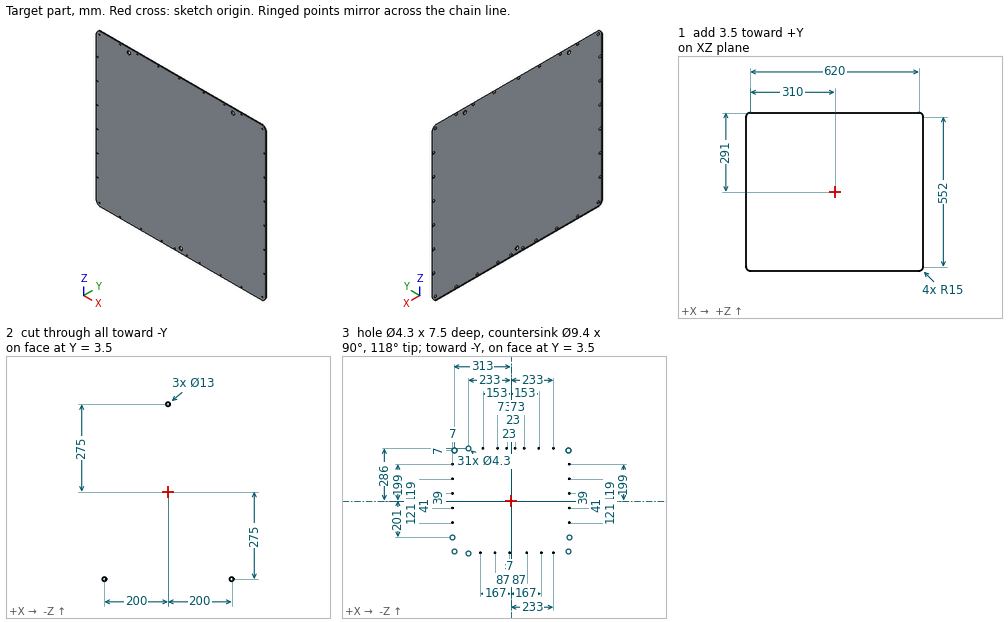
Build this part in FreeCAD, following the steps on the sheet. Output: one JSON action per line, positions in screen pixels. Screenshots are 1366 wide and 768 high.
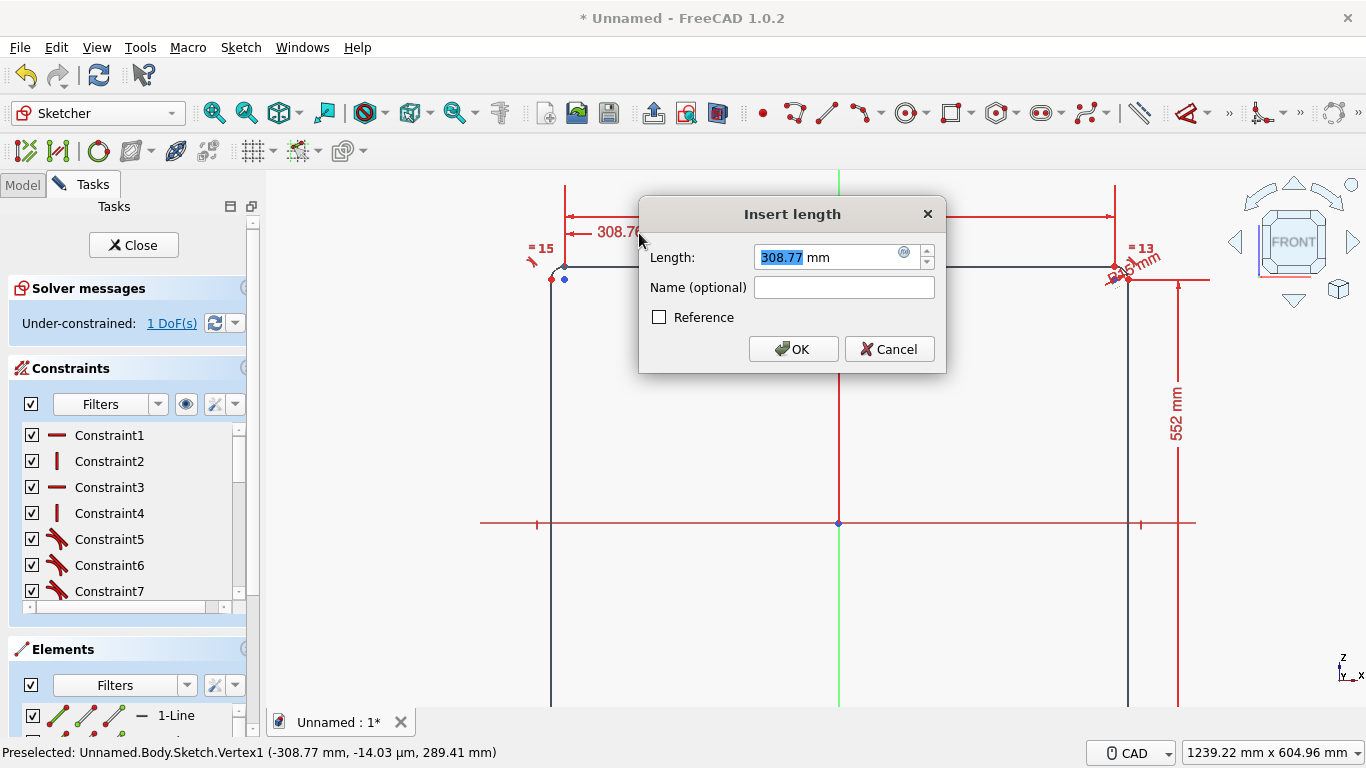
{"action": "type", "text": "310"}
{"action": "key", "text": "Return"}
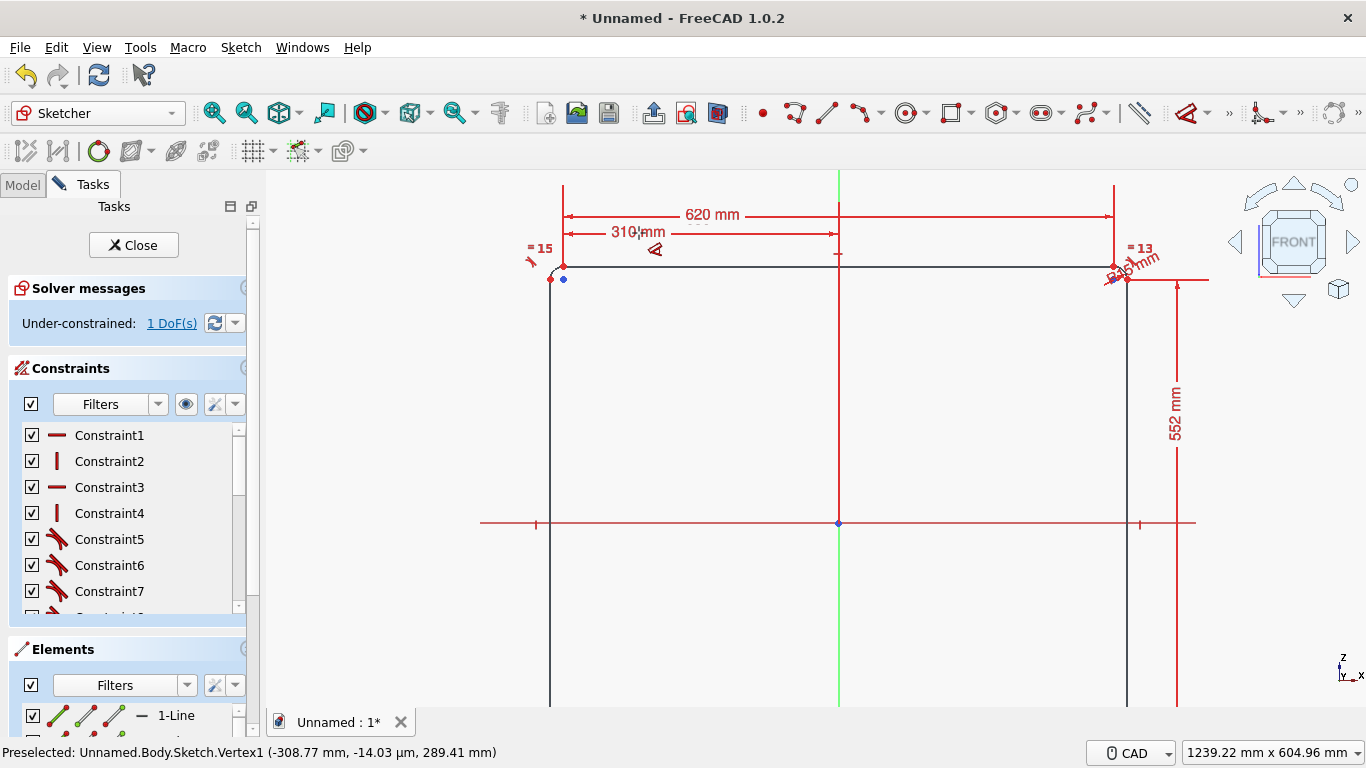
{"action": "left_click", "coordinate": [563, 267]}
{"action": "left_click", "coordinate": [529, 395]}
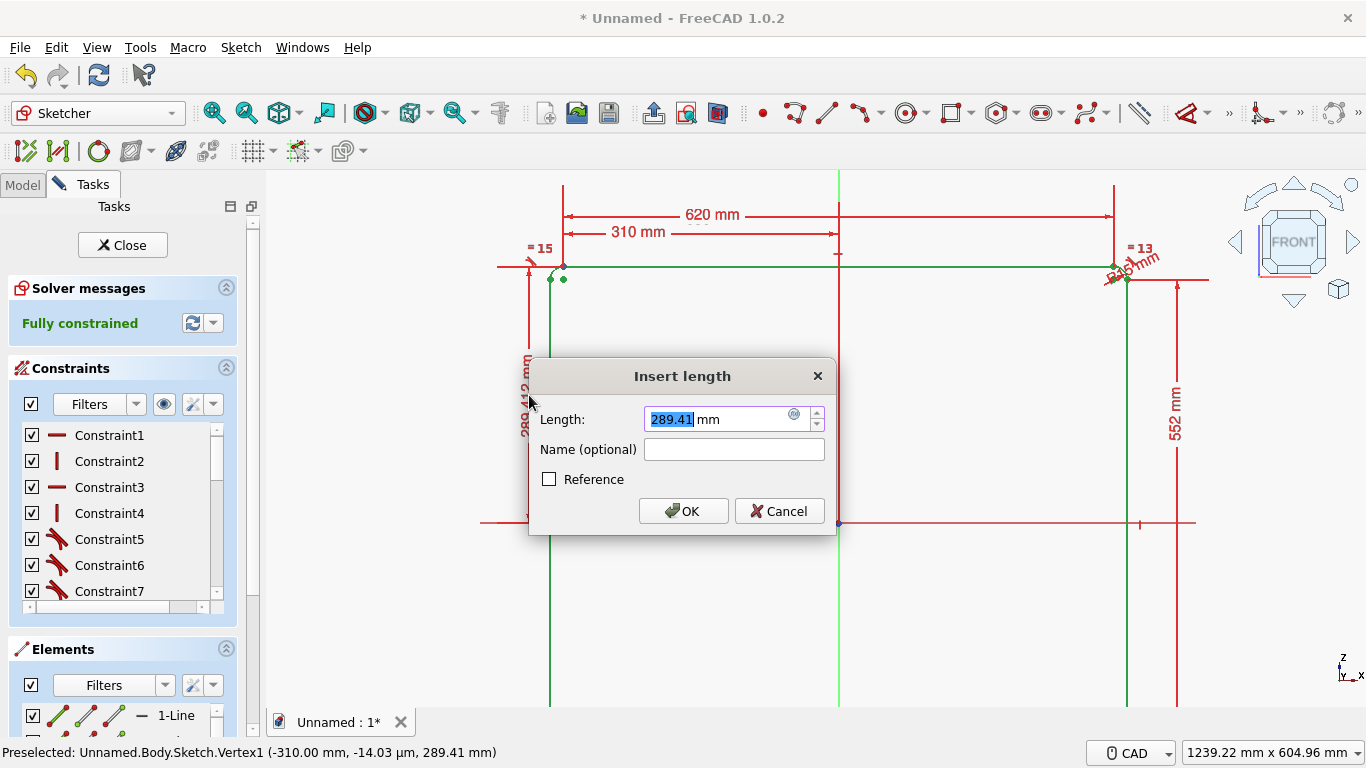
{"action": "type", "text": "291"}
{"action": "key", "text": "Return"}
{"action": "key", "text": "Escape"}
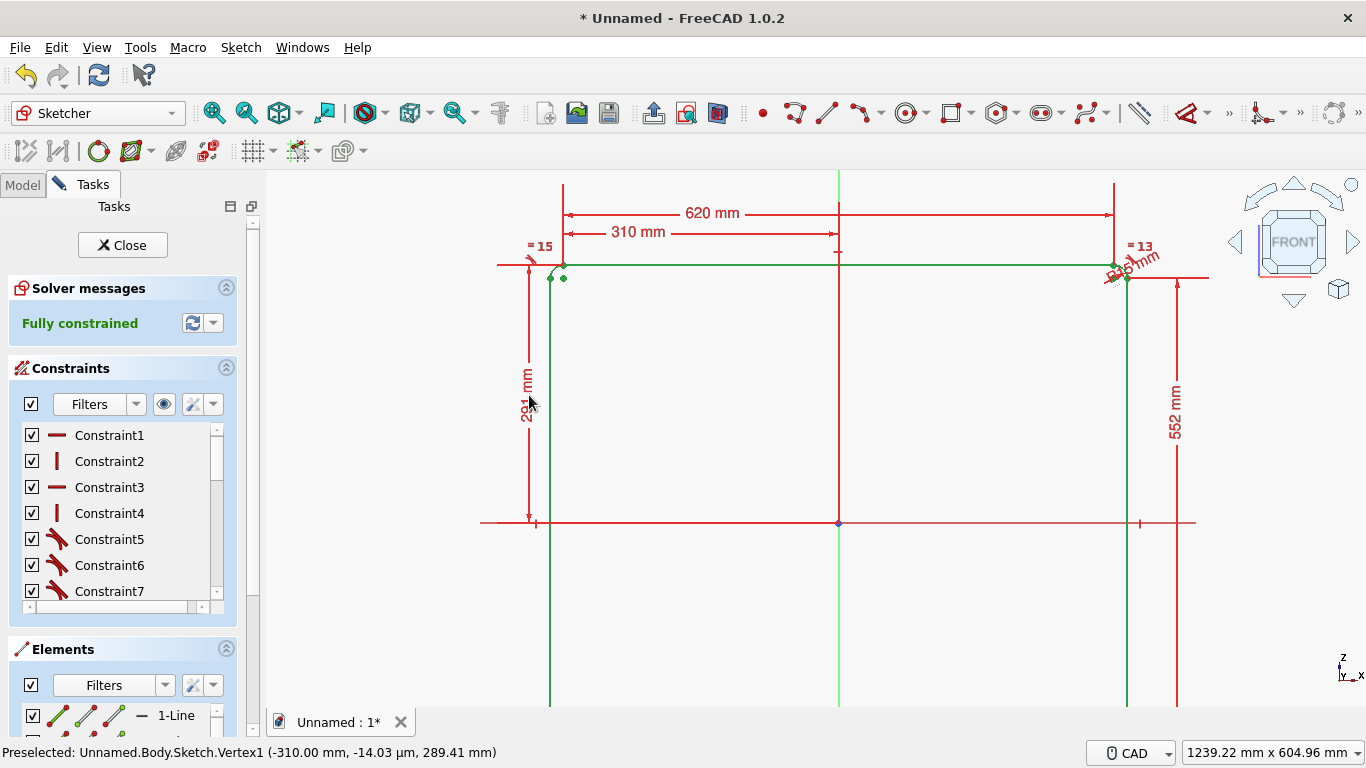
{"action": "left_click", "coordinate": [123, 245]}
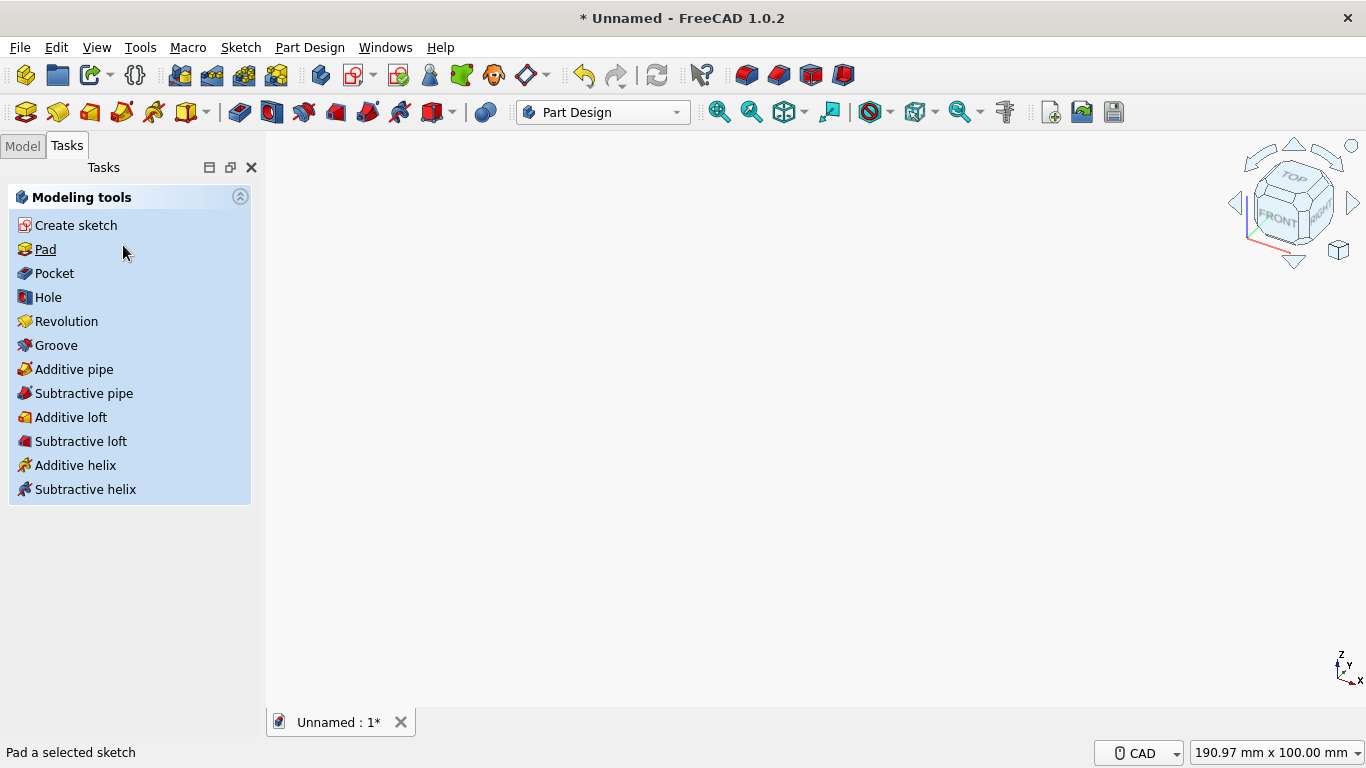
{"action": "left_click", "coordinate": [26, 112]}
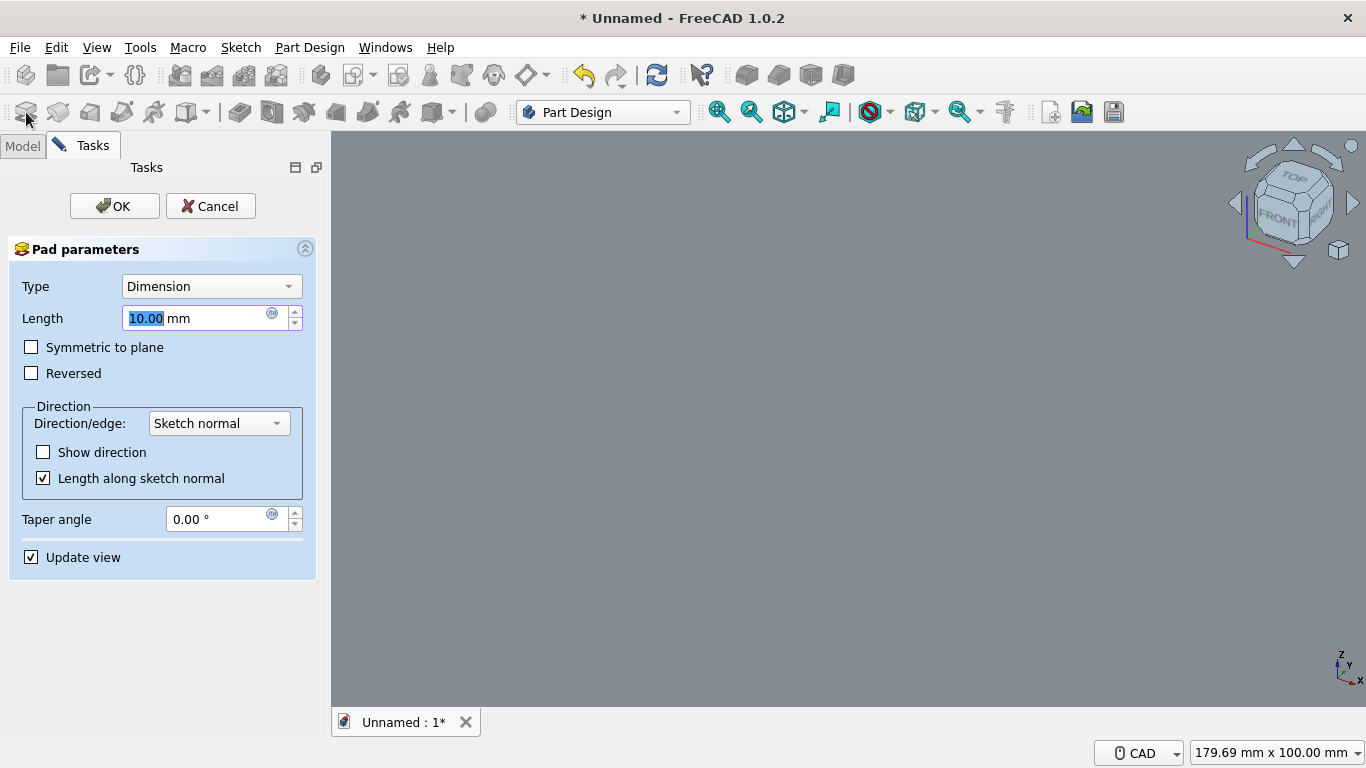
{"action": "type", "text": "3.5"}
{"action": "key", "text": "Tab"}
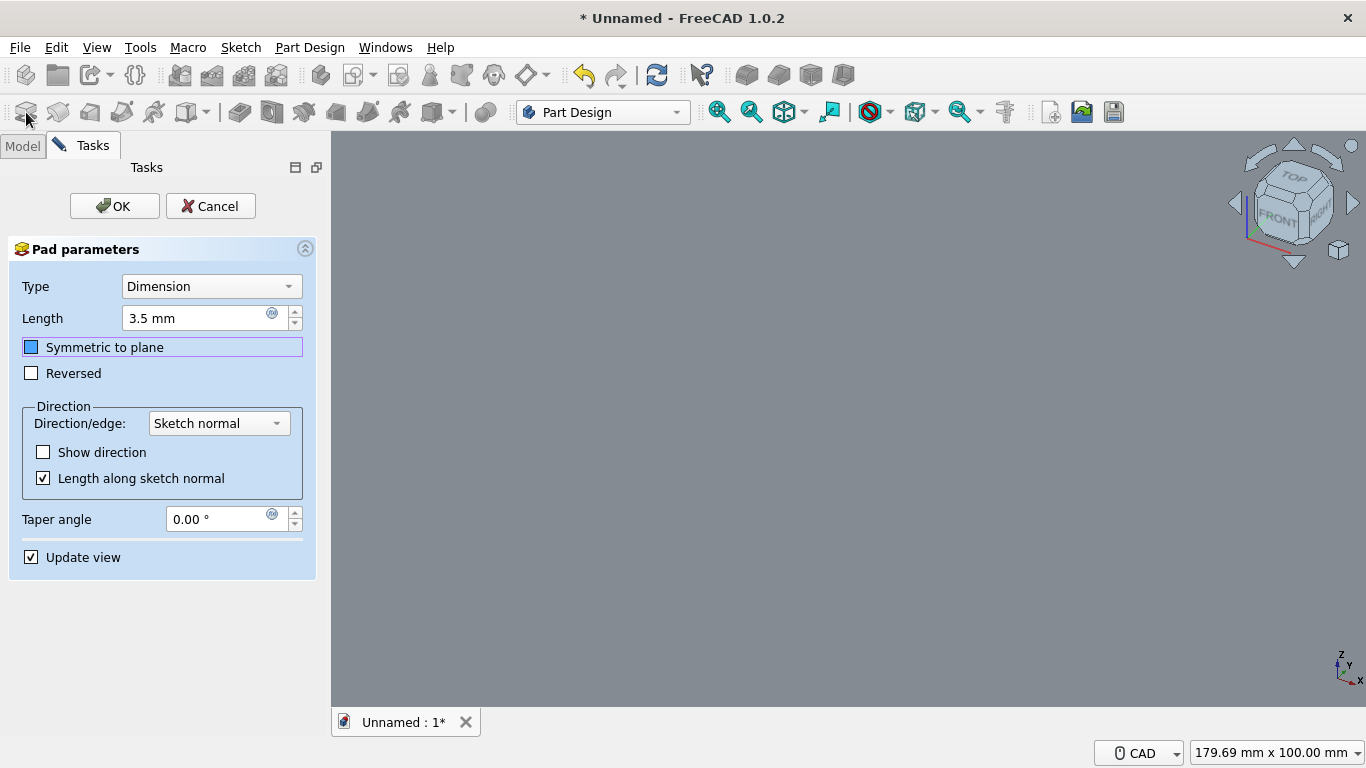
{"action": "left_click", "coordinate": [30, 373]}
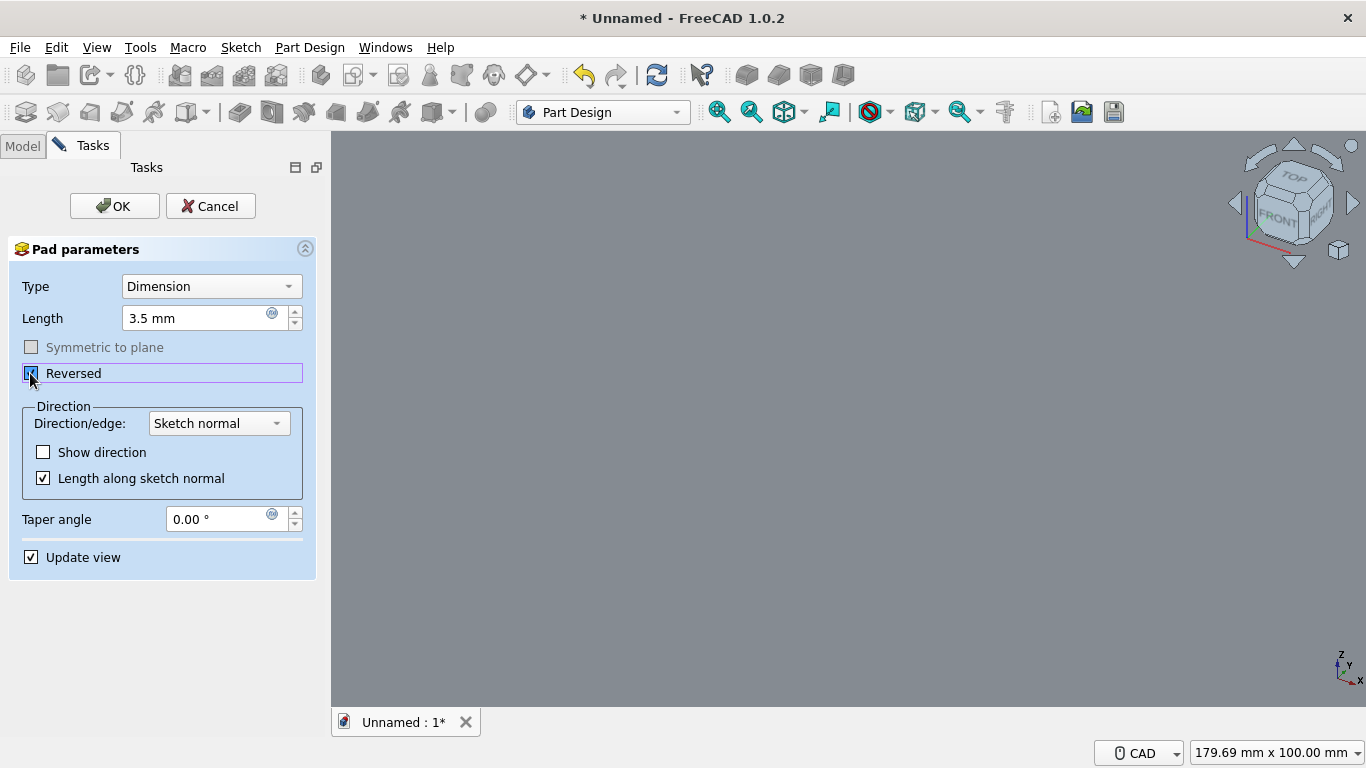
{"action": "left_click", "coordinate": [115, 206]}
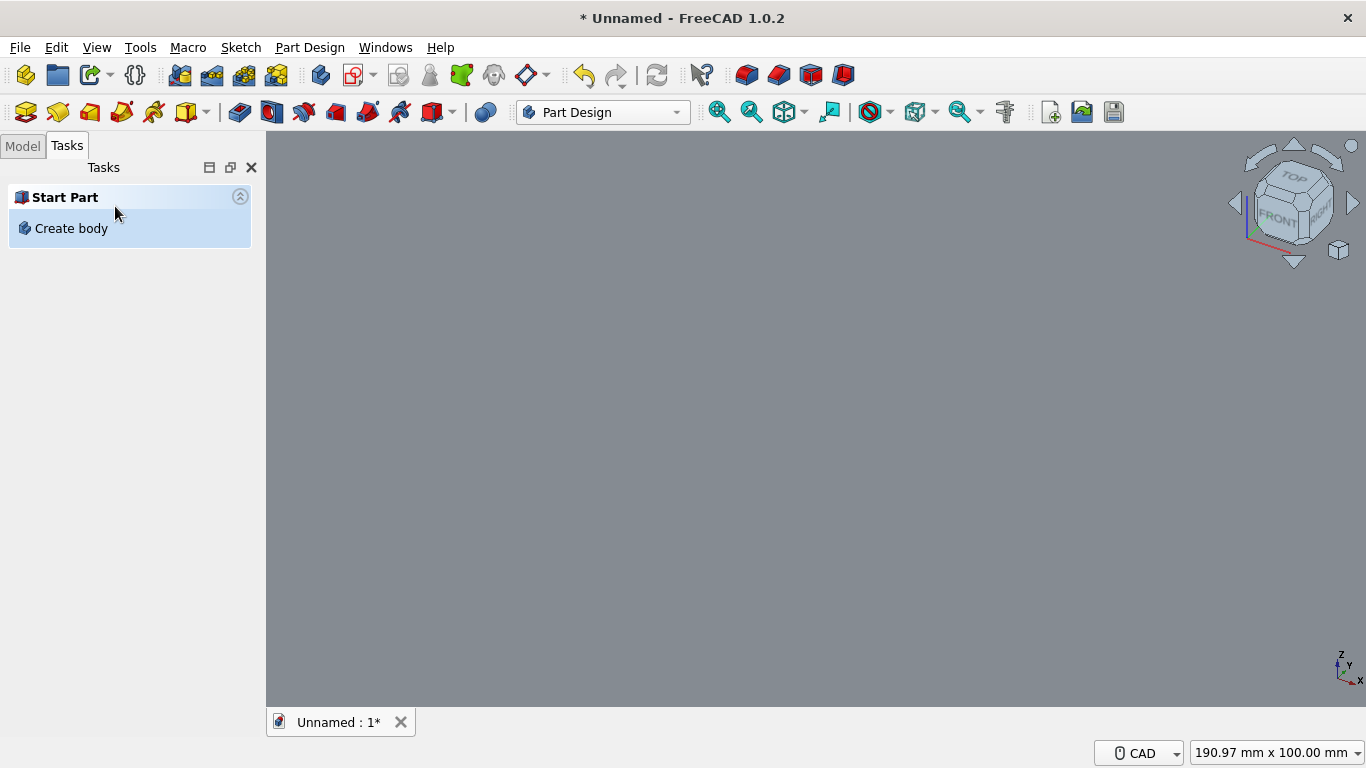
{"action": "left_click", "coordinate": [720, 112]}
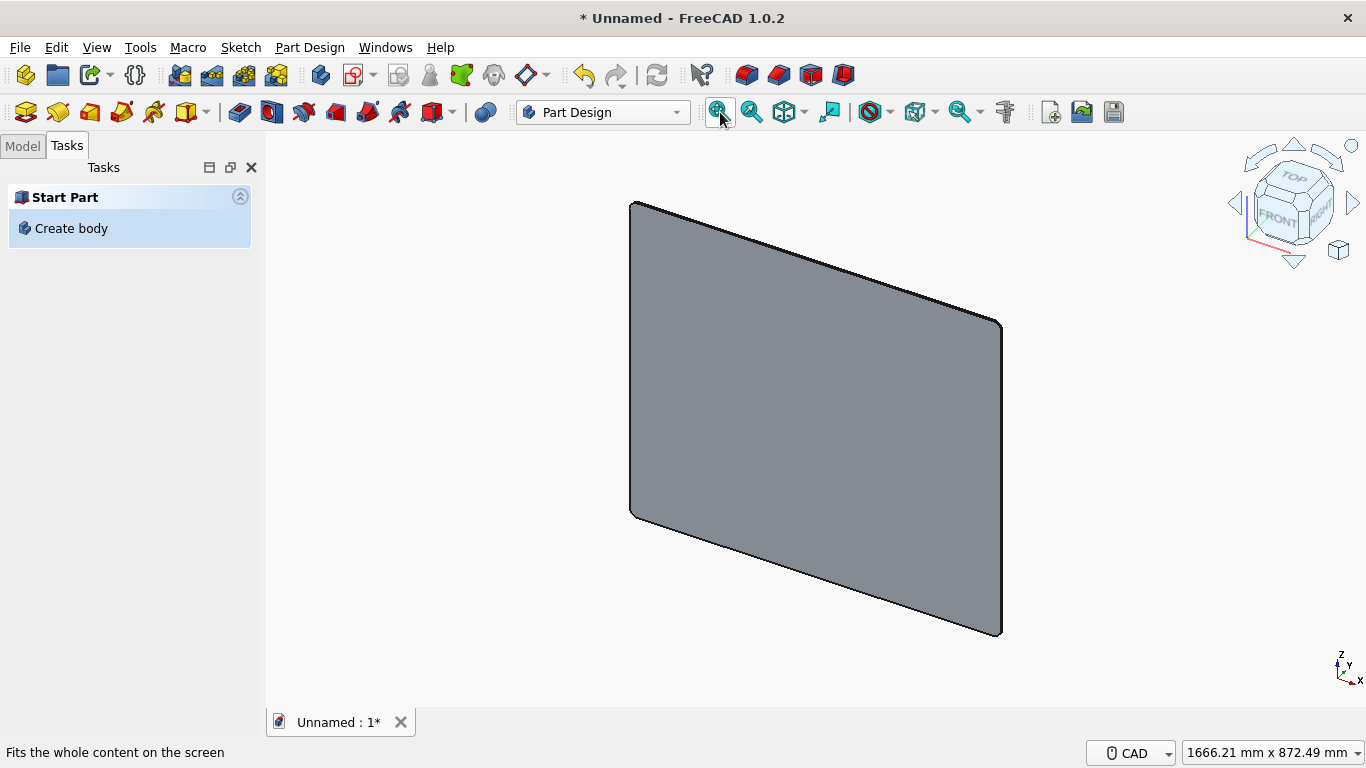
{"action": "key", "text": "4"}